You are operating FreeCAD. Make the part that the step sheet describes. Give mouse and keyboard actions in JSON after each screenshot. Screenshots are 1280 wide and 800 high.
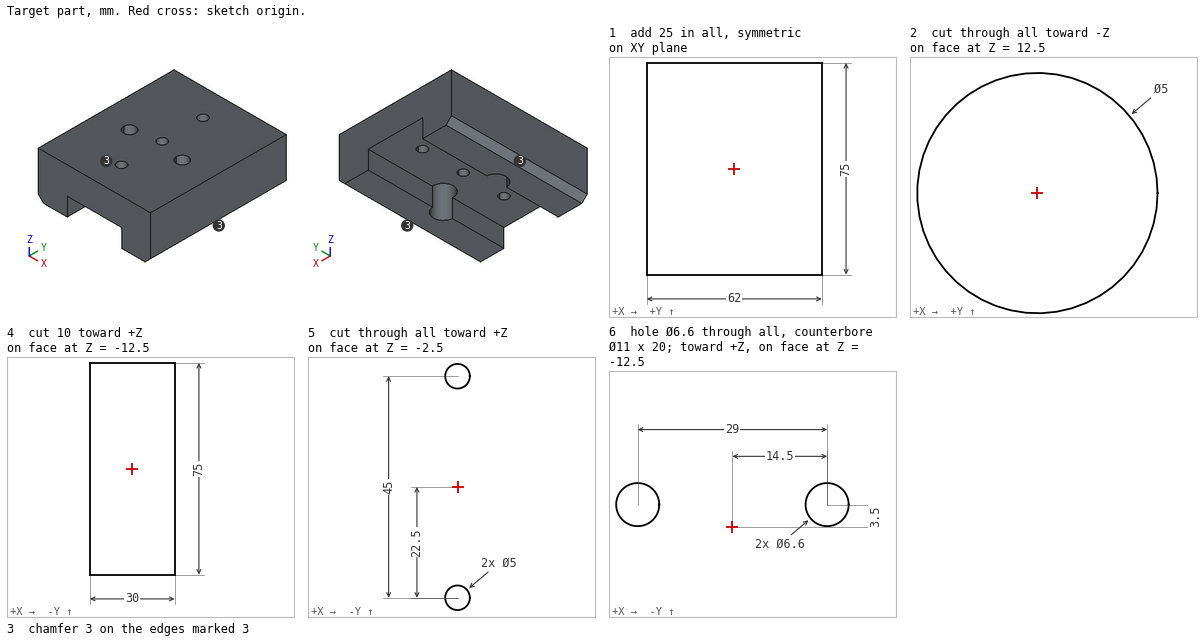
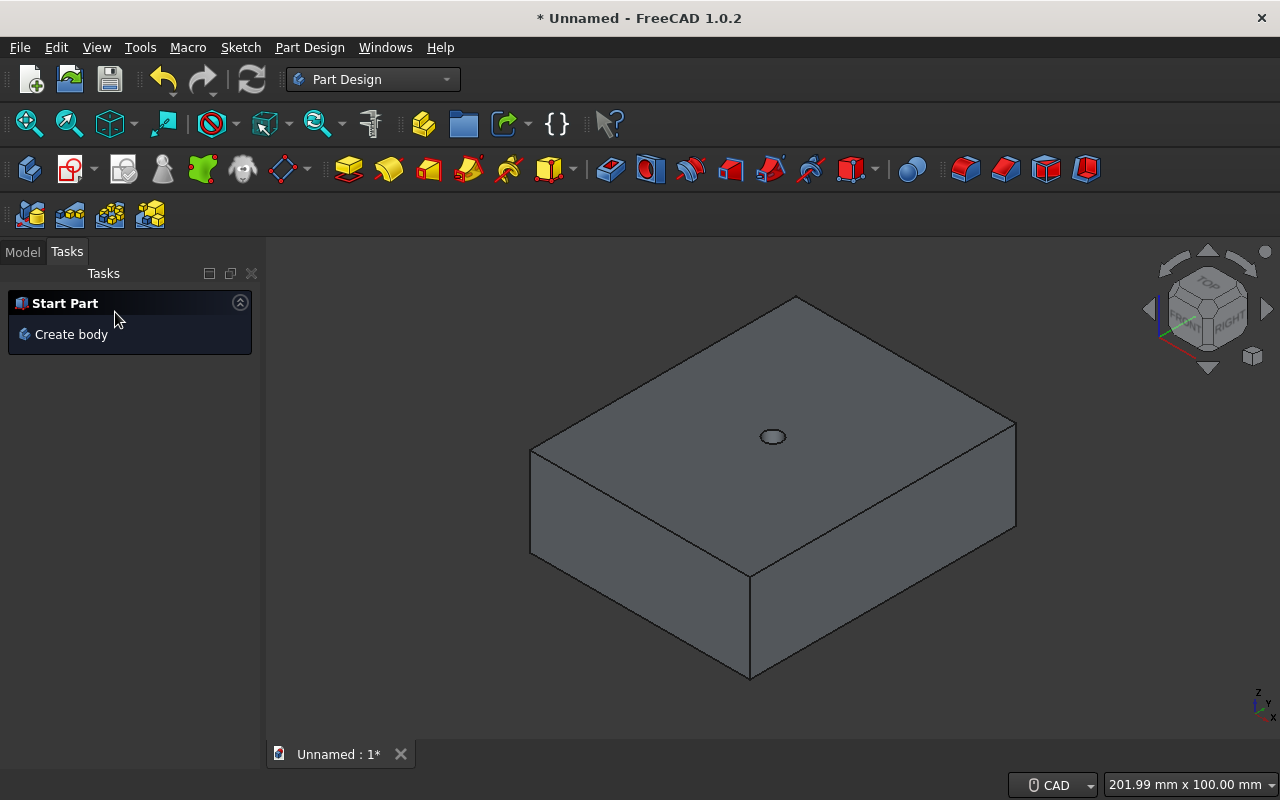
{"action": "key", "text": "2"}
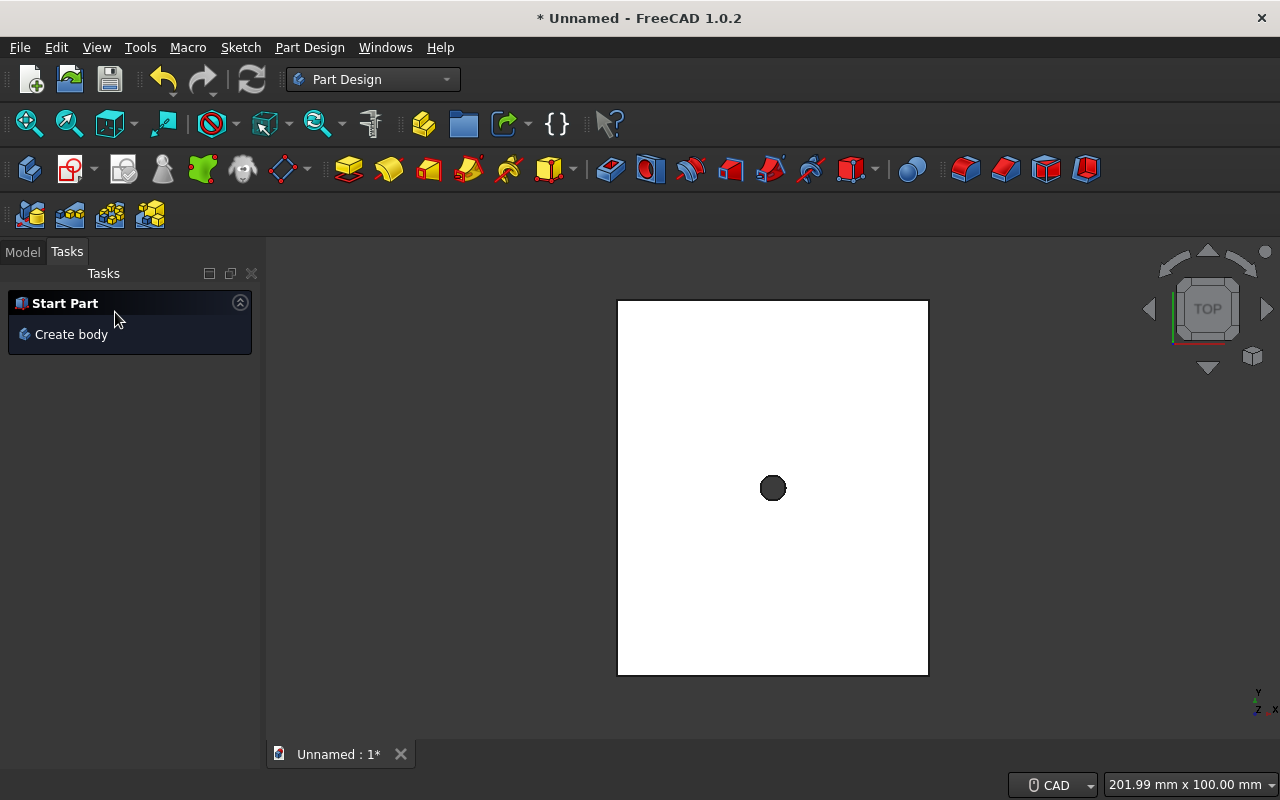
{"action": "key", "text": "1"}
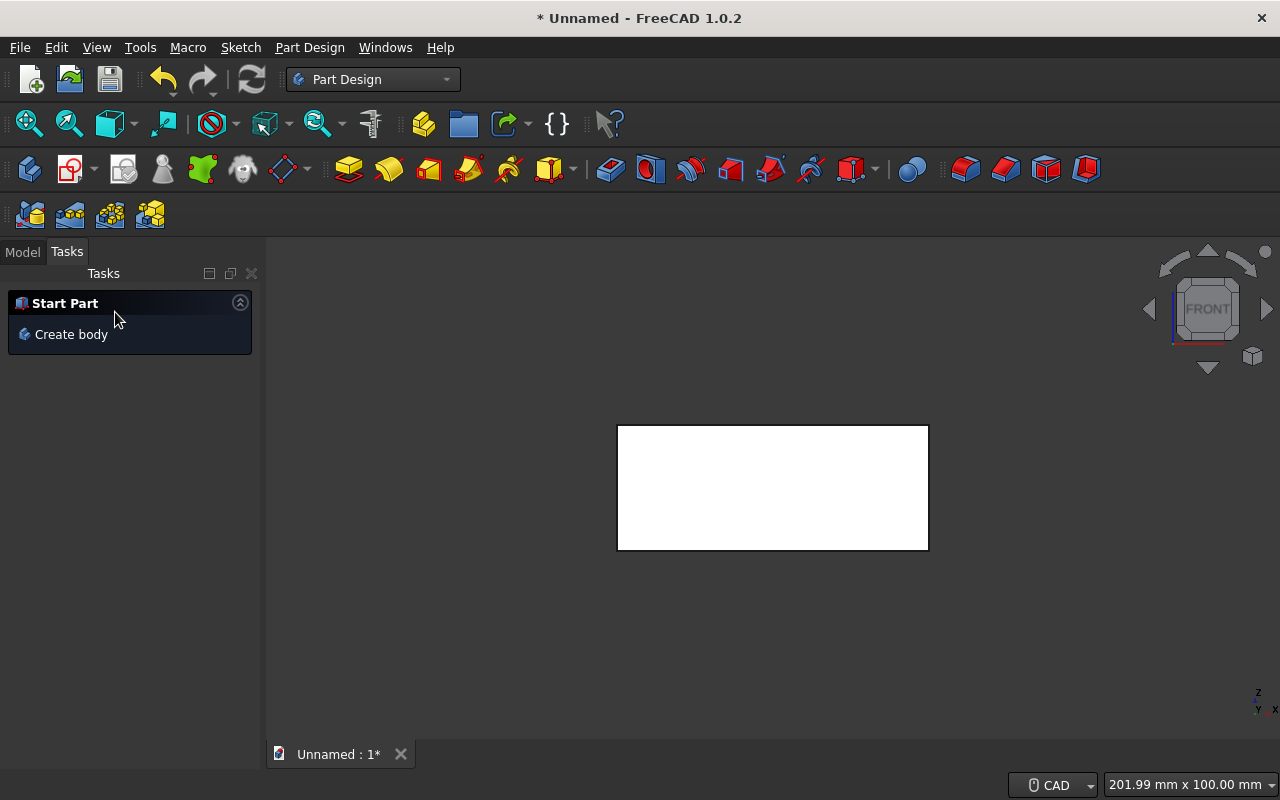
{"action": "key", "text": "v f"}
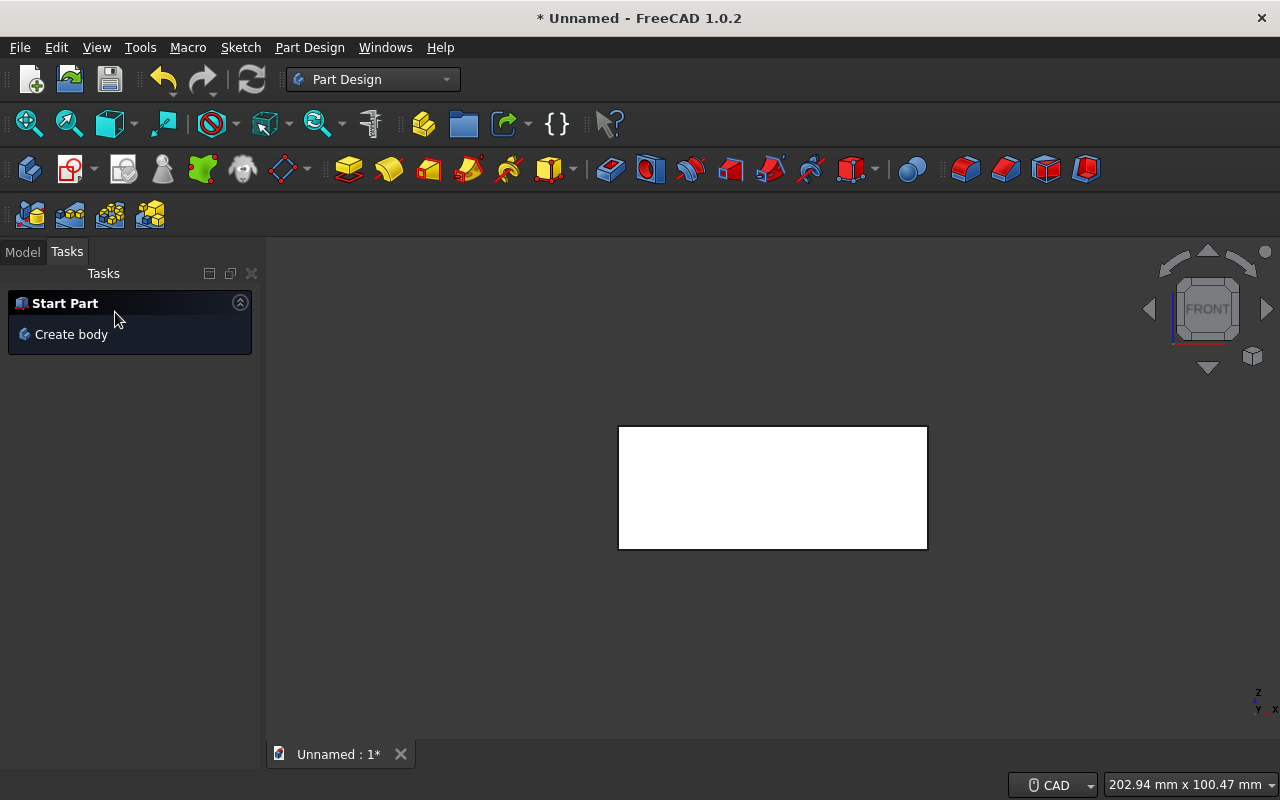
{"action": "key", "text": "3"}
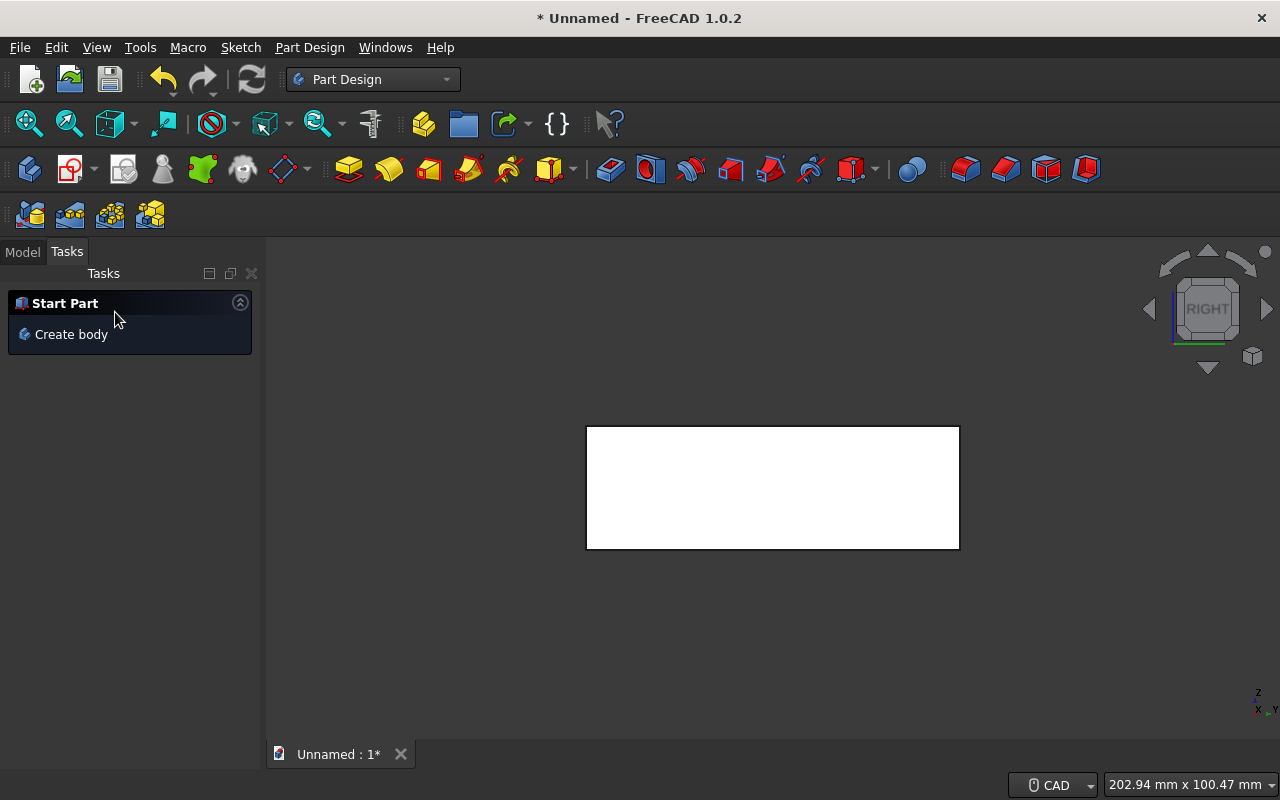
{"action": "key", "text": "v f"}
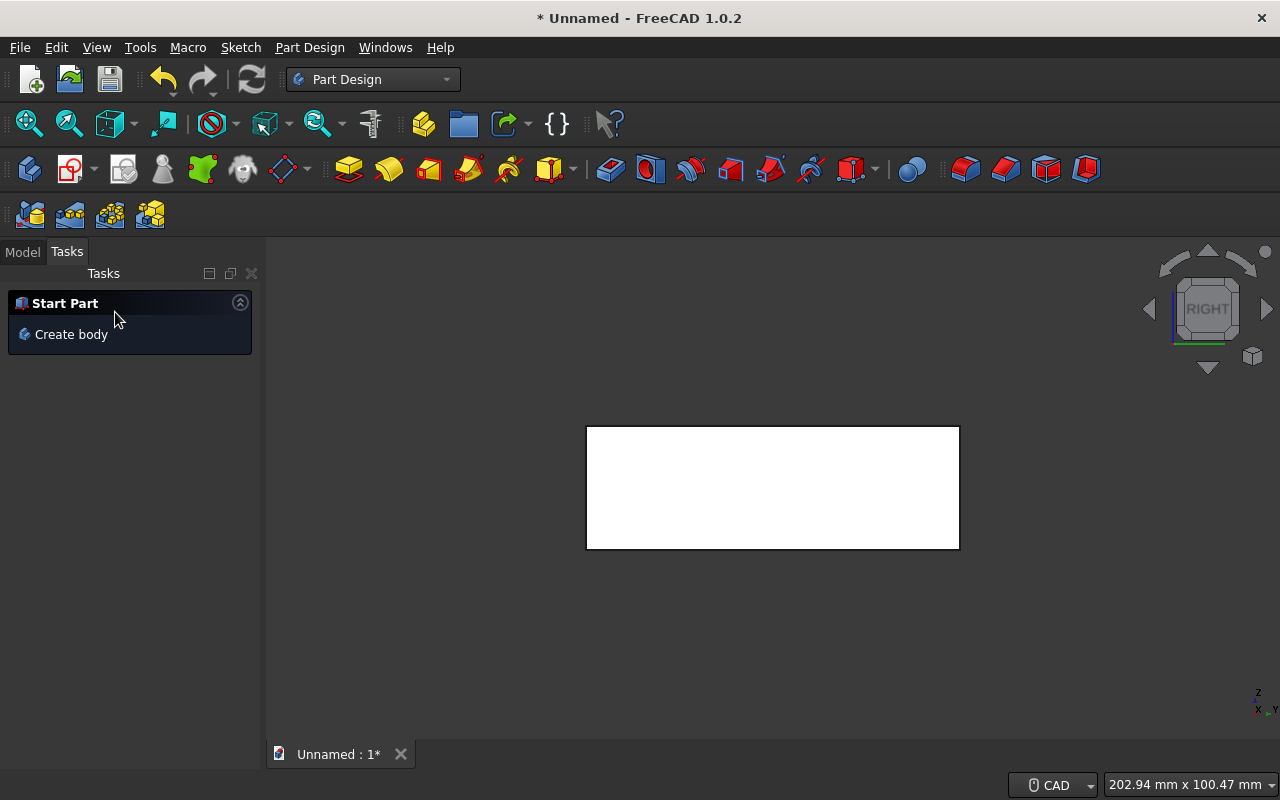
{"action": "left_click", "coordinate": [773, 549]}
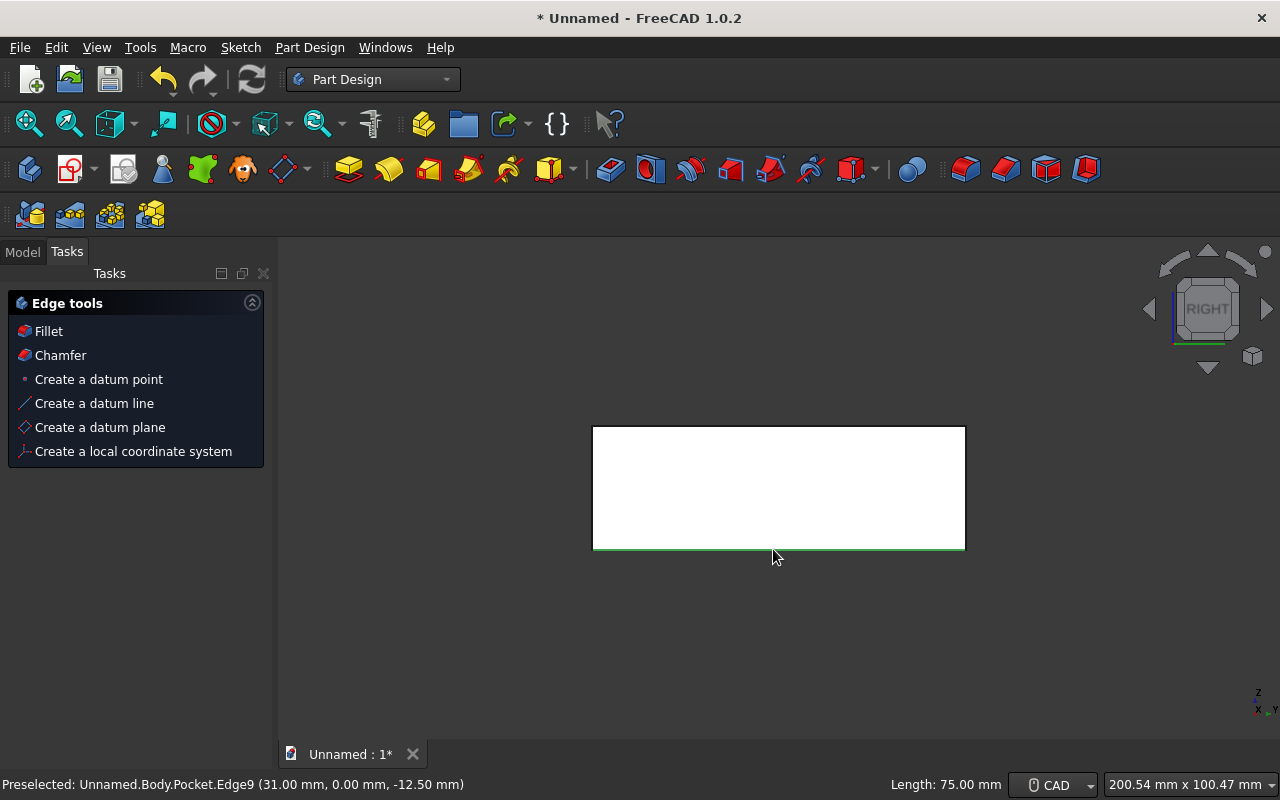
{"action": "key", "text": "5"}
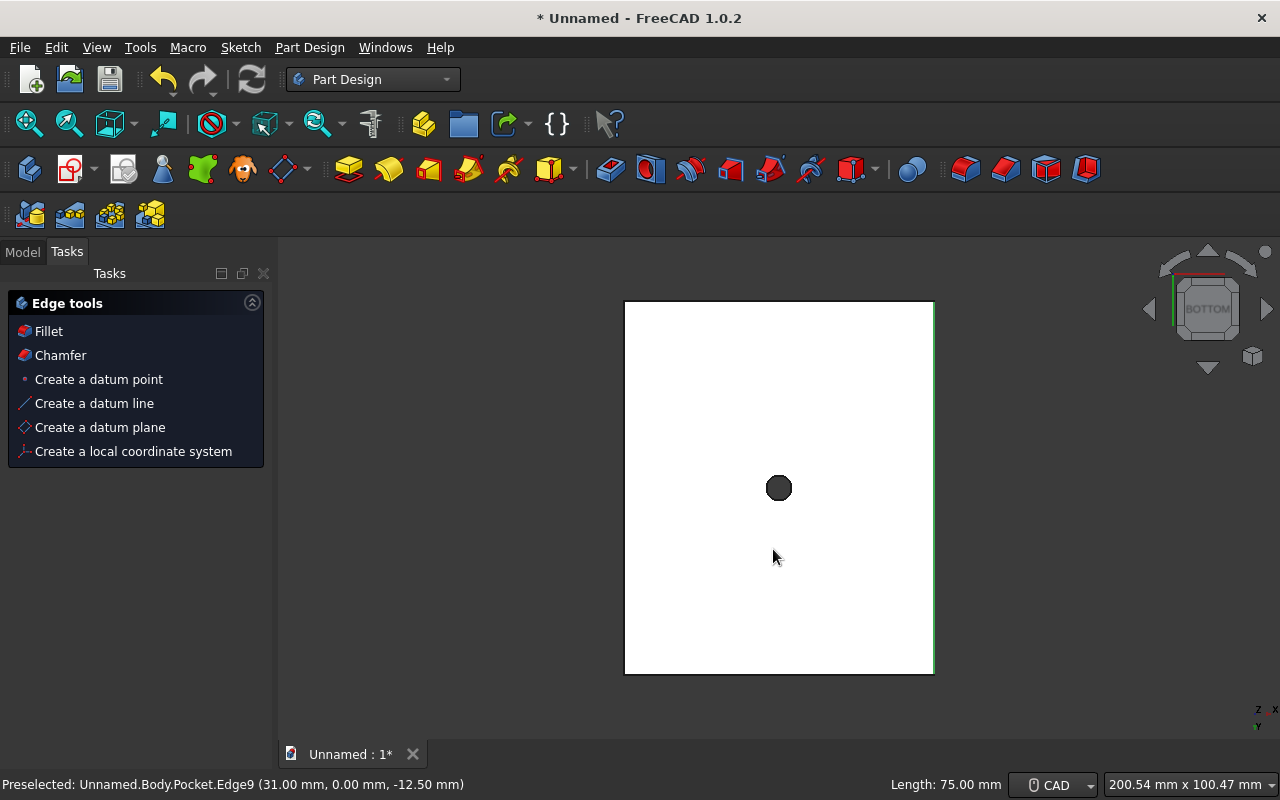
{"action": "left_click", "coordinate": [624, 487], "text": "ctrl"}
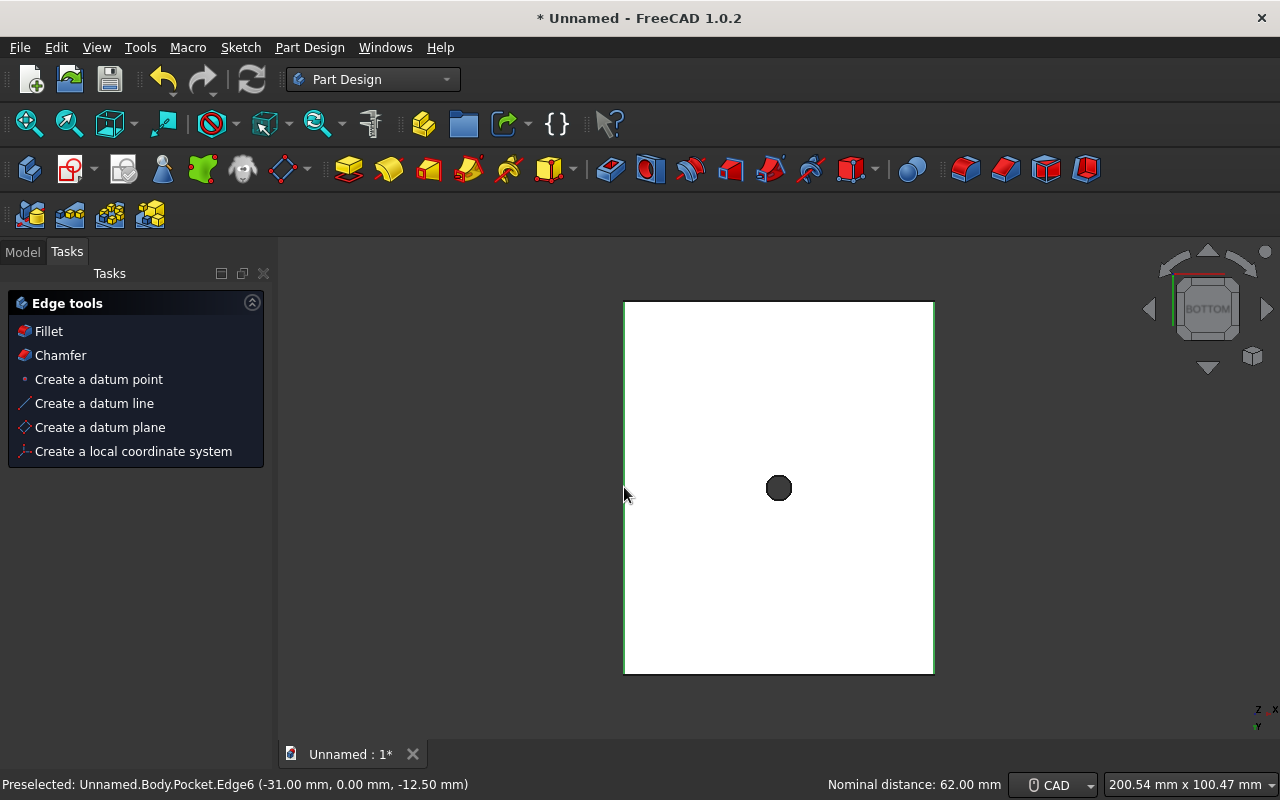
{"action": "left_click", "coordinate": [1006, 170]}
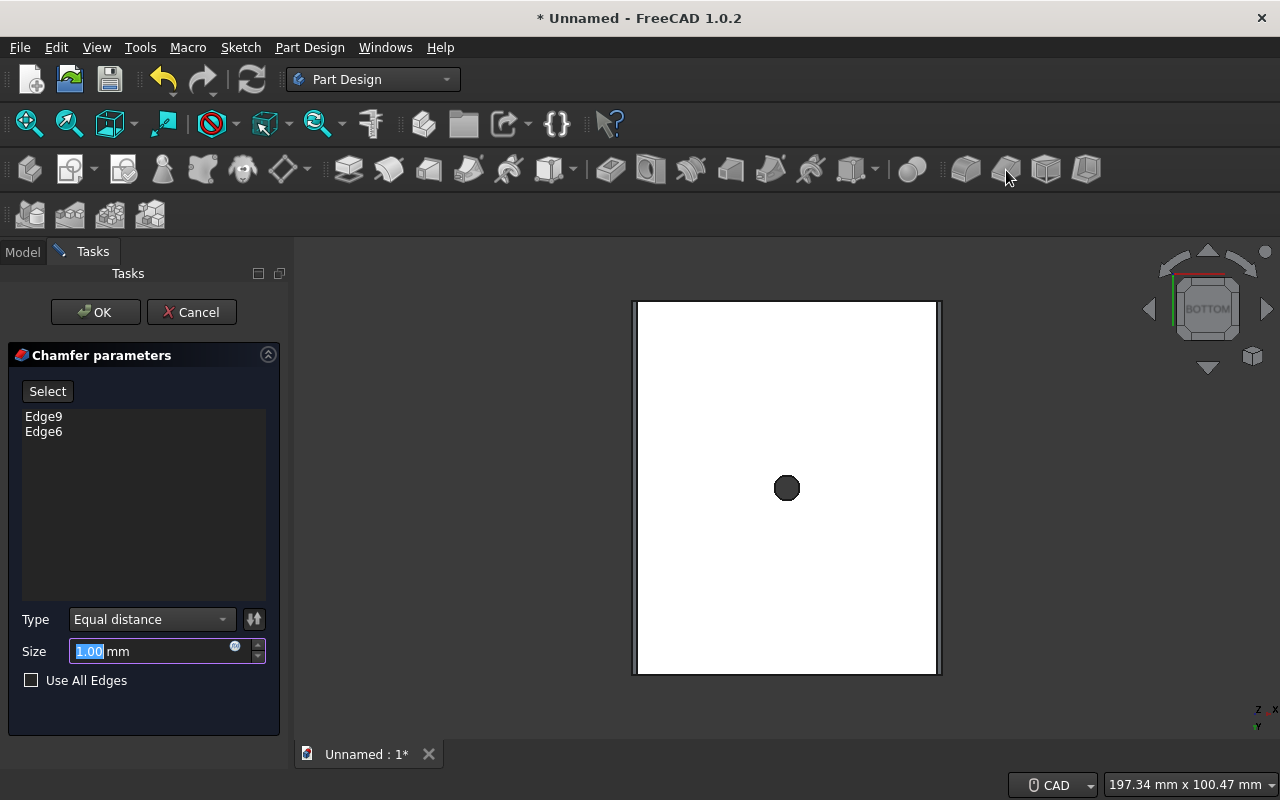
{"action": "type", "text": "3"}
{"action": "key", "text": "Tab"}